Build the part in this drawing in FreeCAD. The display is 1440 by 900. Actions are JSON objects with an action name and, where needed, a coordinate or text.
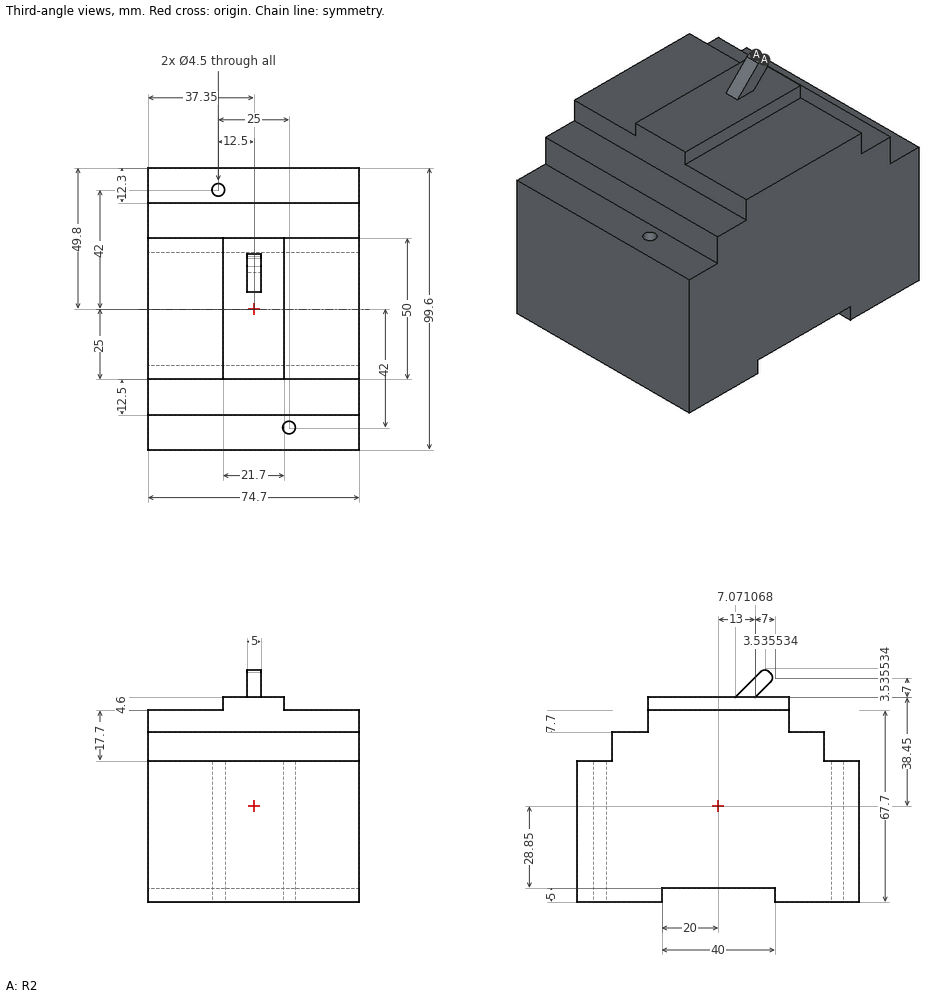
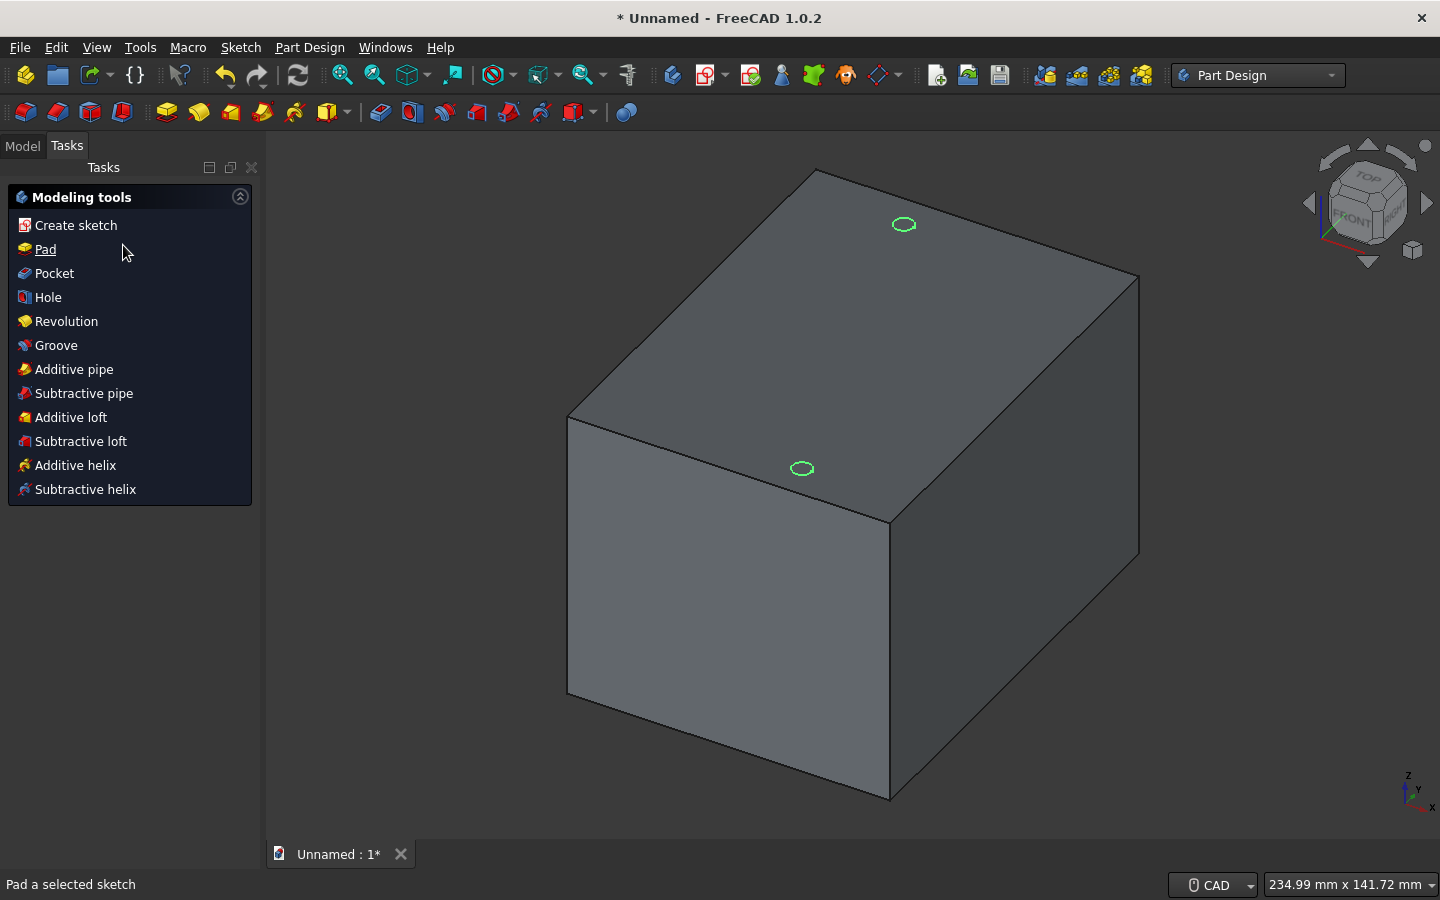
{"action": "left_click", "coordinate": [414, 112]}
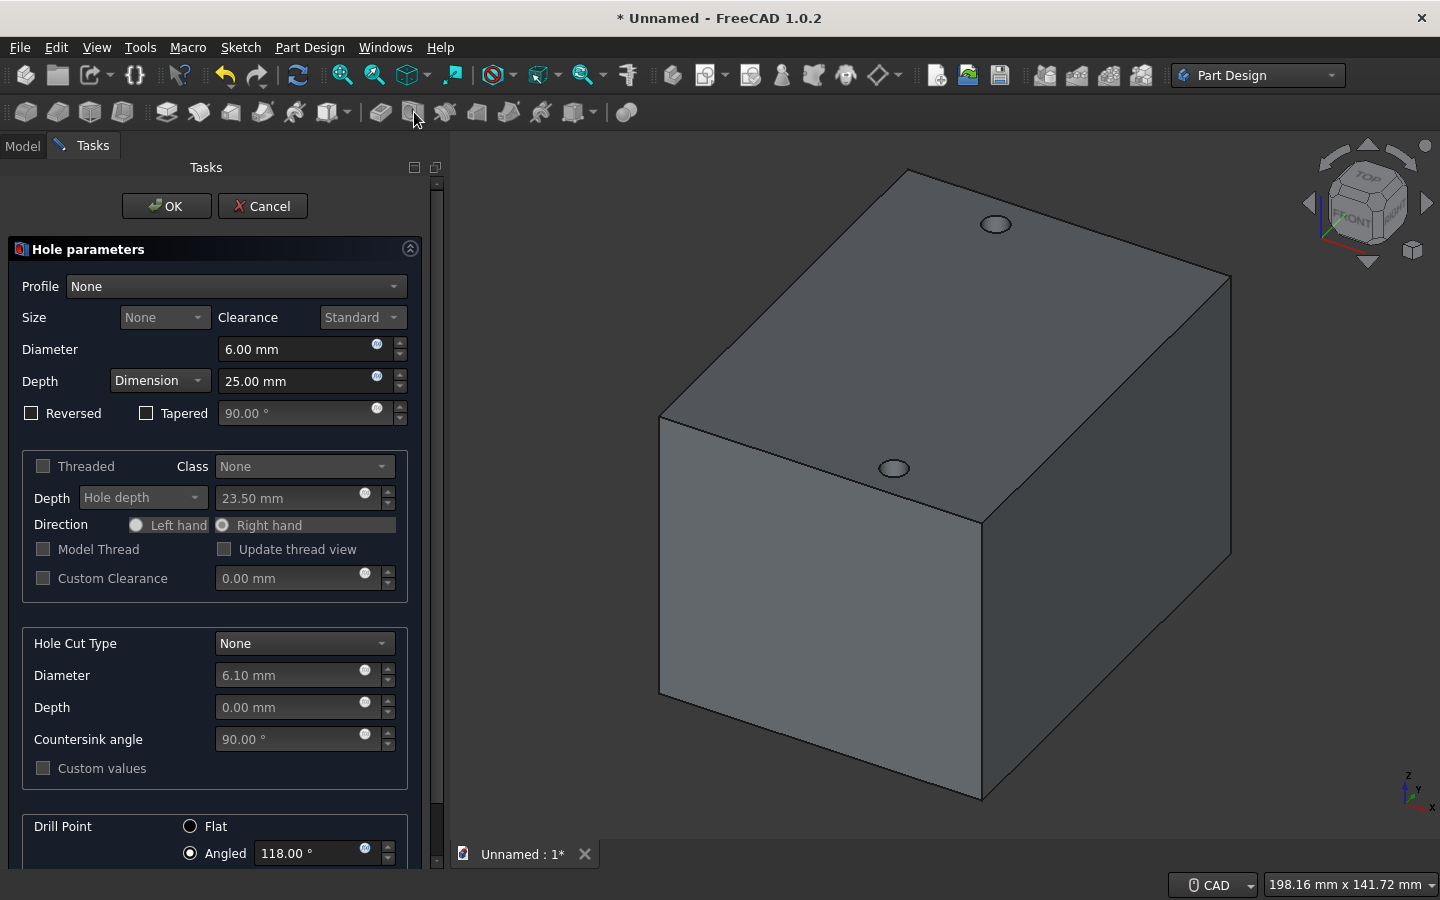
{"action": "triple_click", "coordinate": [305, 349]}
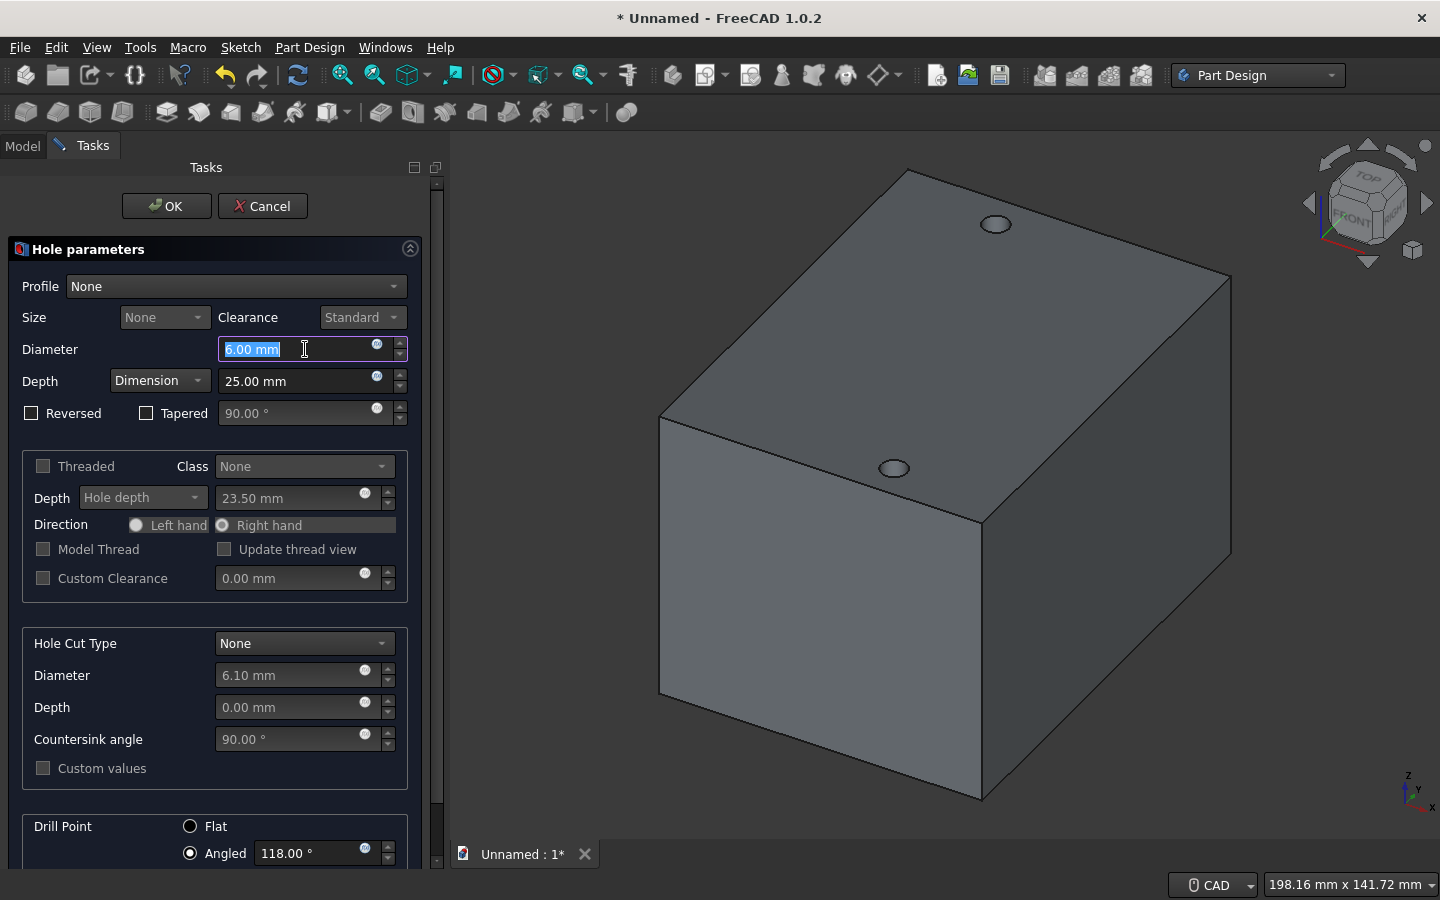
{"action": "type", "text": "4.5"}
{"action": "key", "text": "Tab"}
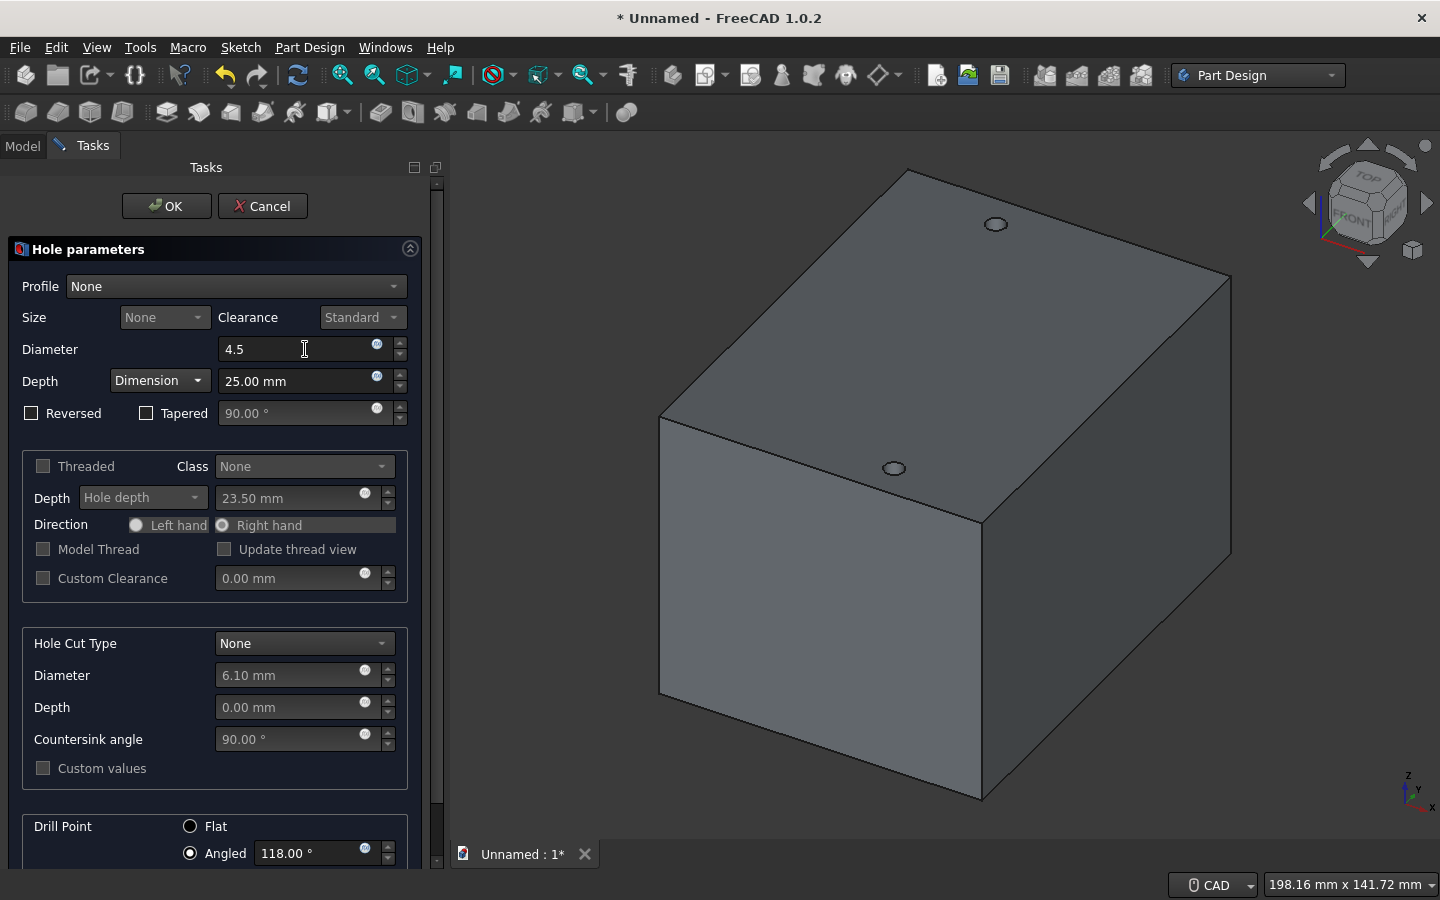
{"action": "left_click", "coordinate": [161, 380]}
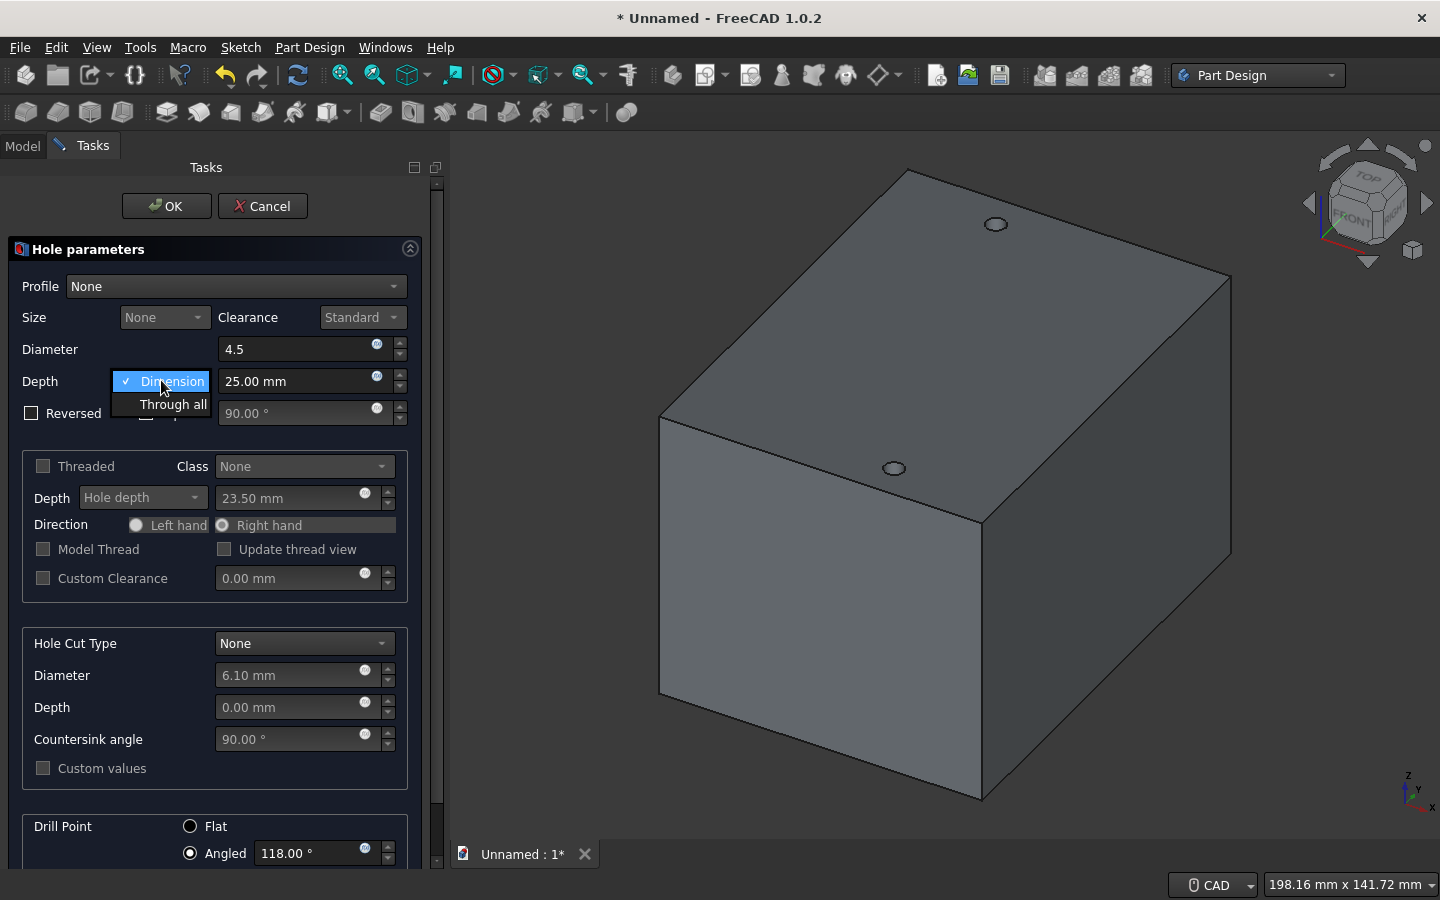
{"action": "left_click", "coordinate": [160, 404]}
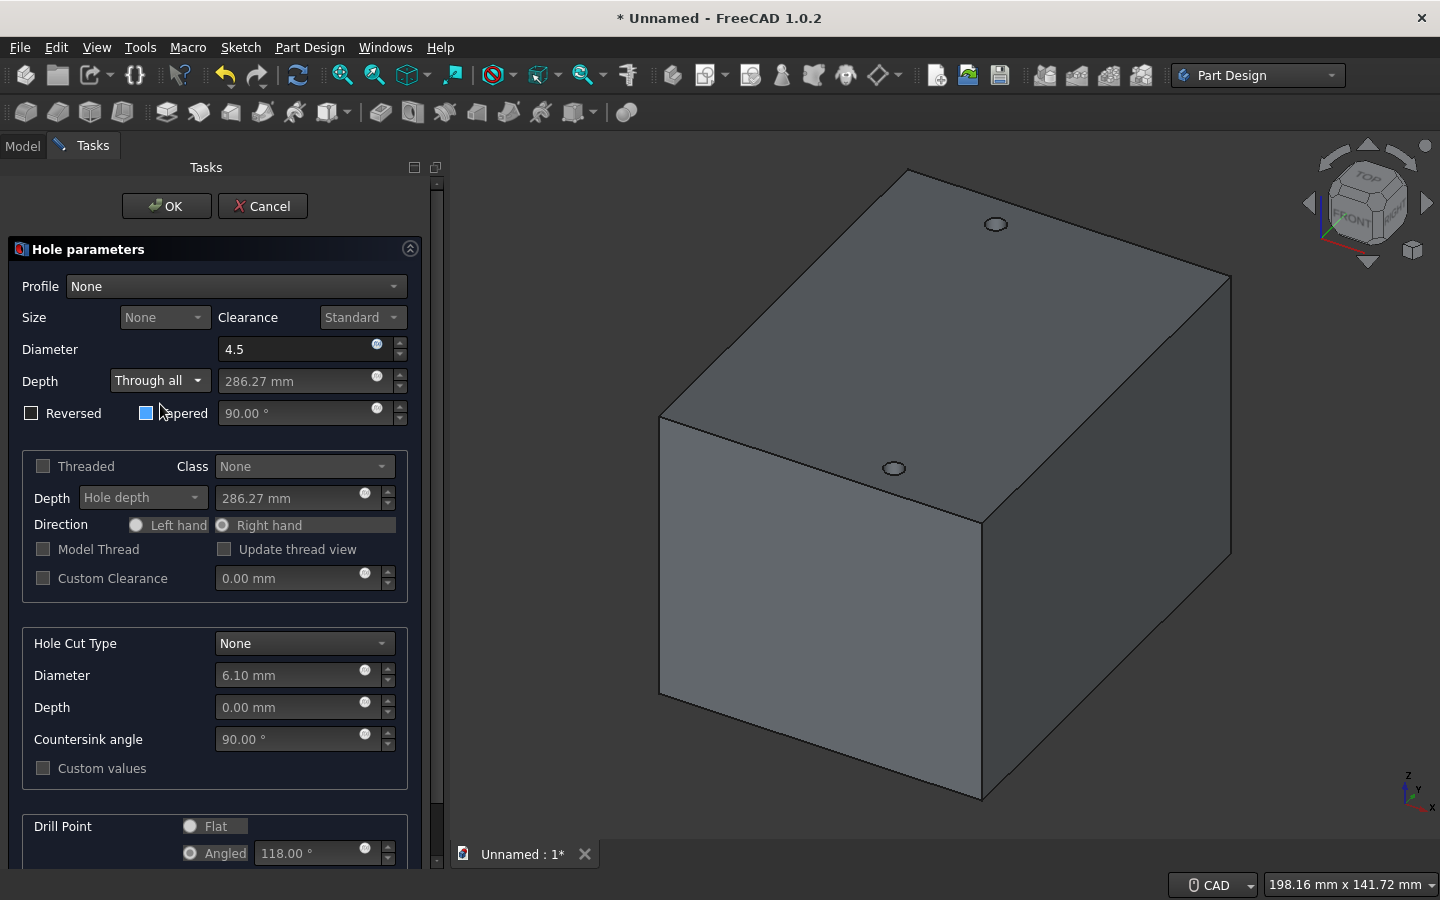
{"action": "left_click", "coordinate": [167, 206]}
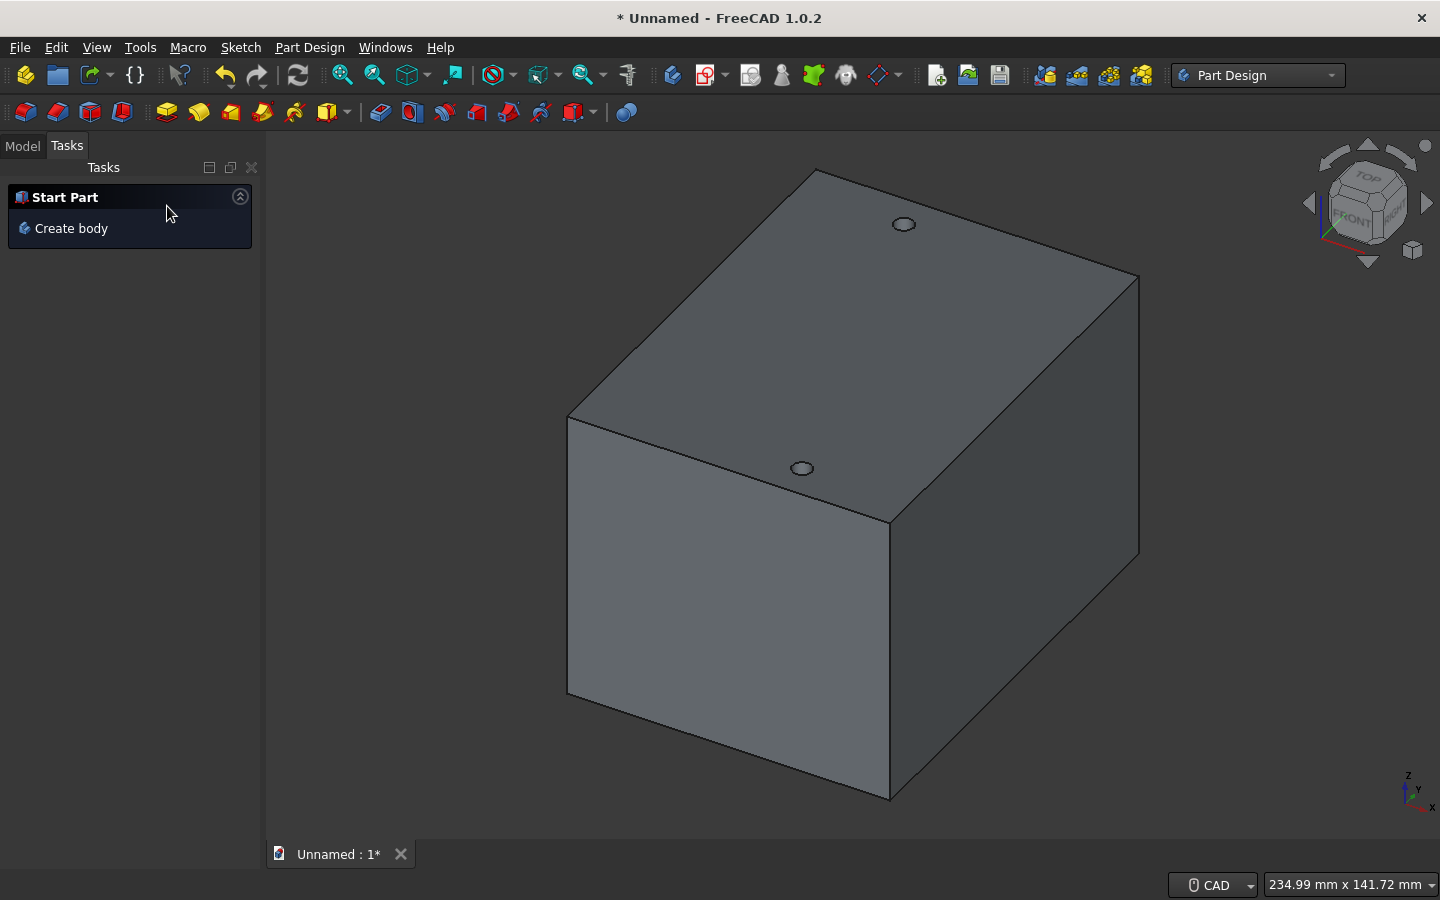
{"action": "left_click", "coordinate": [853, 345]}